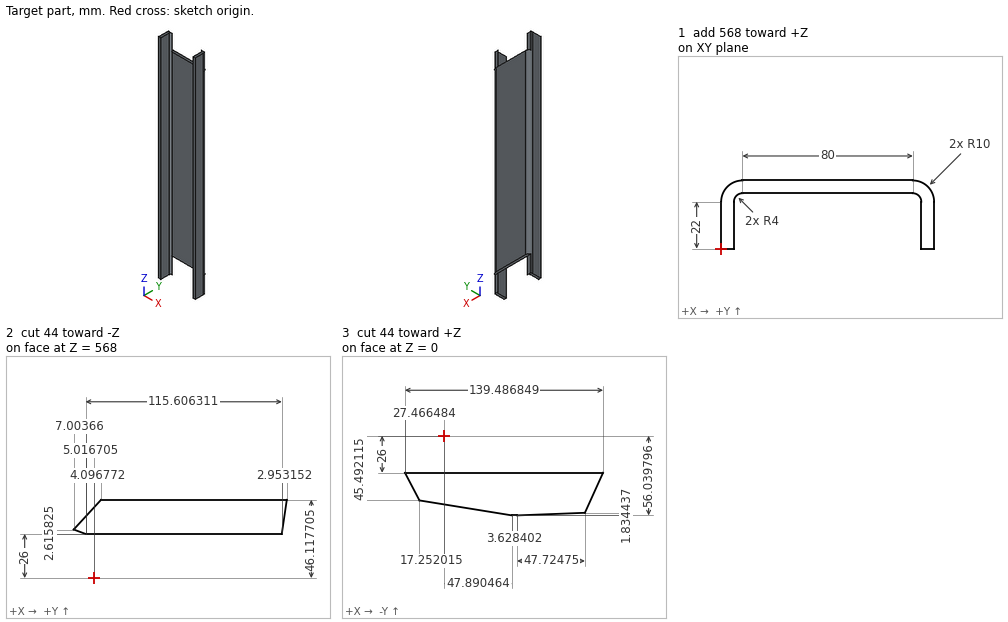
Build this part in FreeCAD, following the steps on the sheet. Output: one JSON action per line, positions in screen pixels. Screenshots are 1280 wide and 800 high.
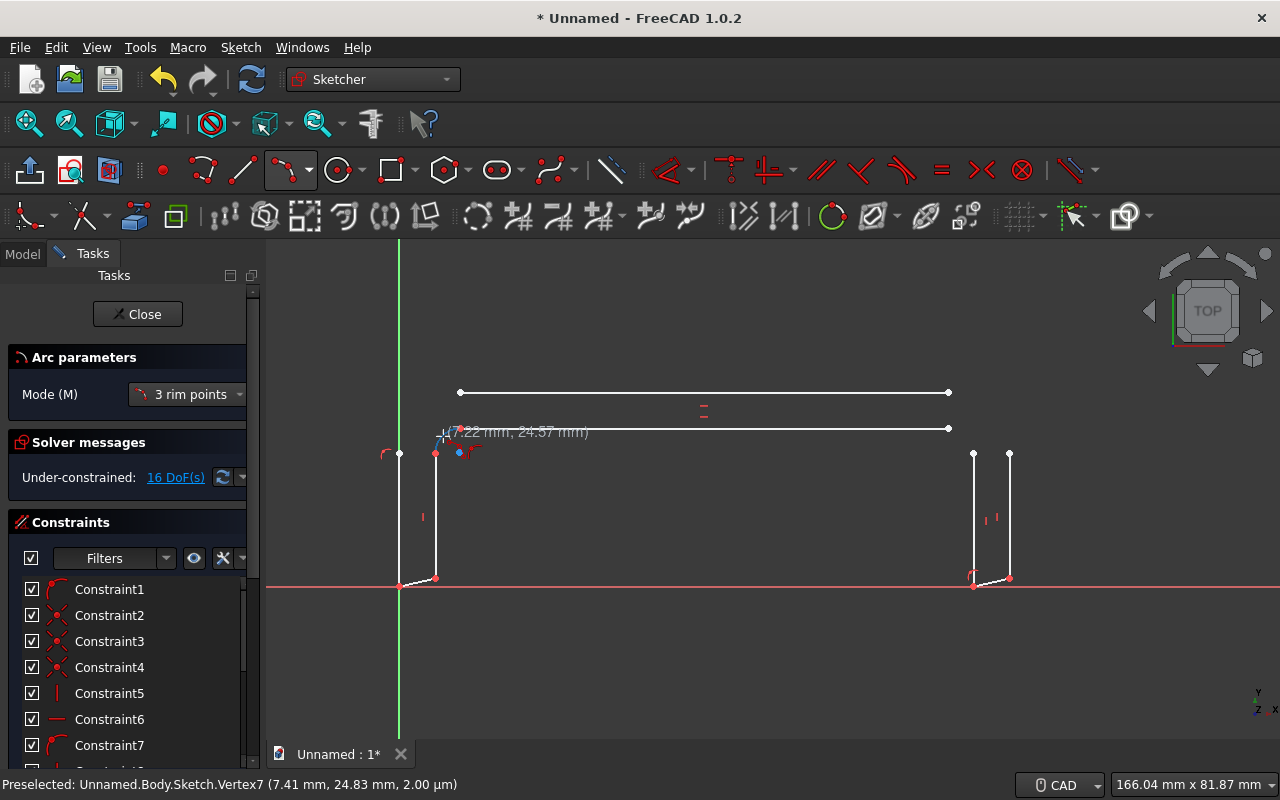
{"action": "left_click", "coordinate": [949, 429]}
{"action": "left_click", "coordinate": [974, 454]}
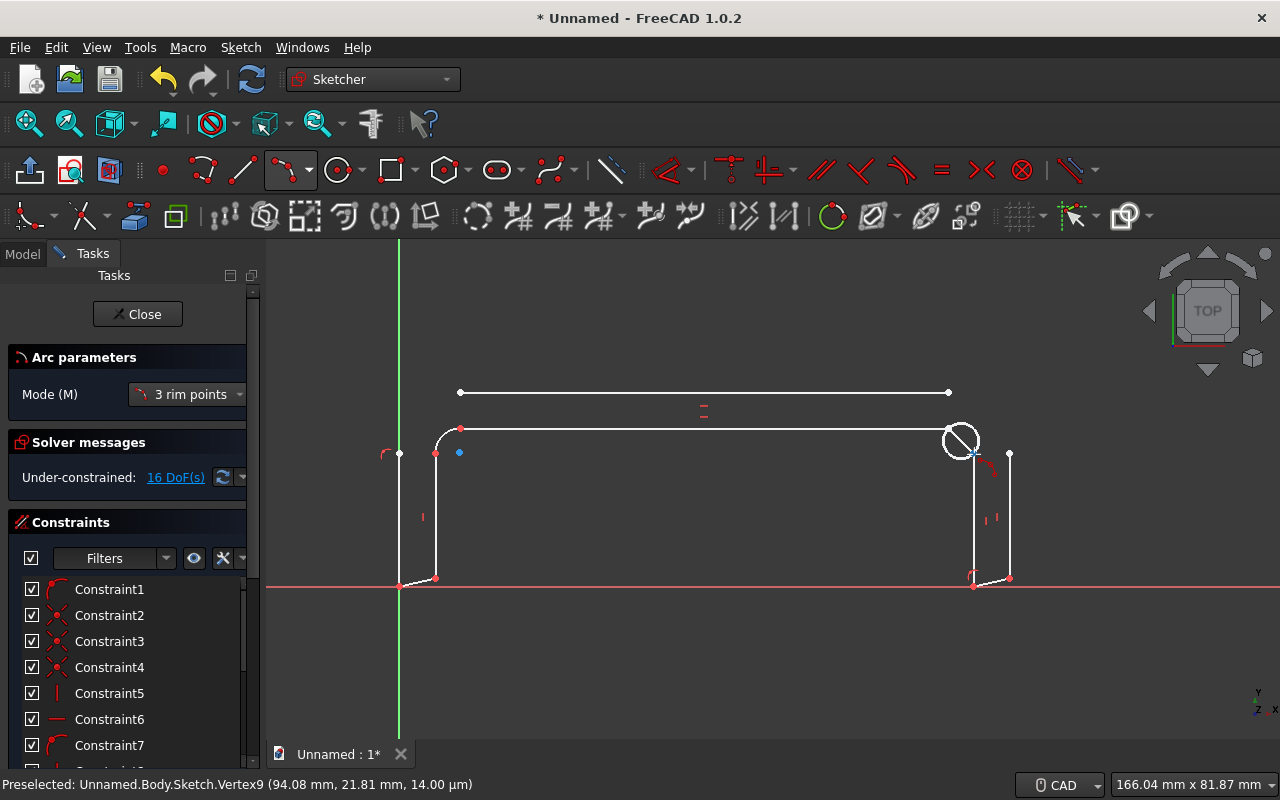
{"action": "scroll", "coordinate": [966, 435], "scroll_direction": "up", "scroll_amount": 4}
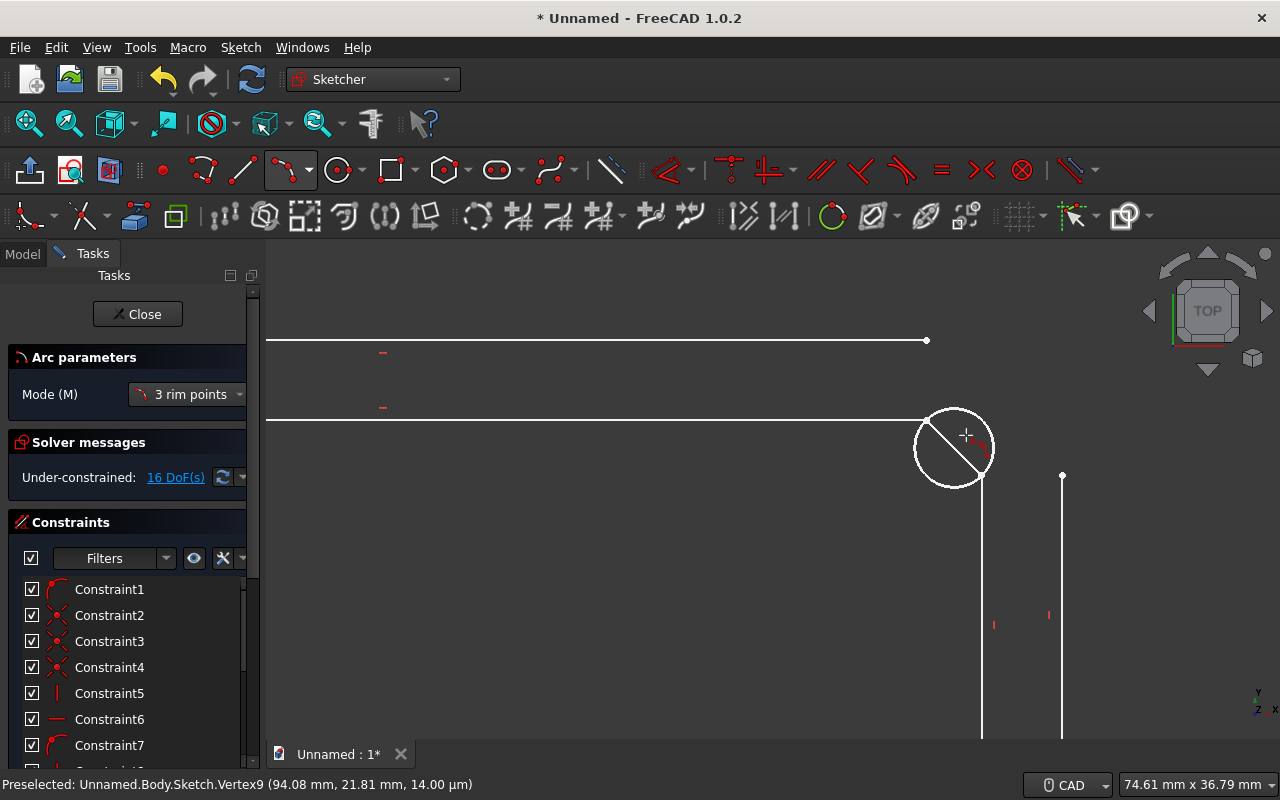
{"action": "left_click", "coordinate": [965, 435]}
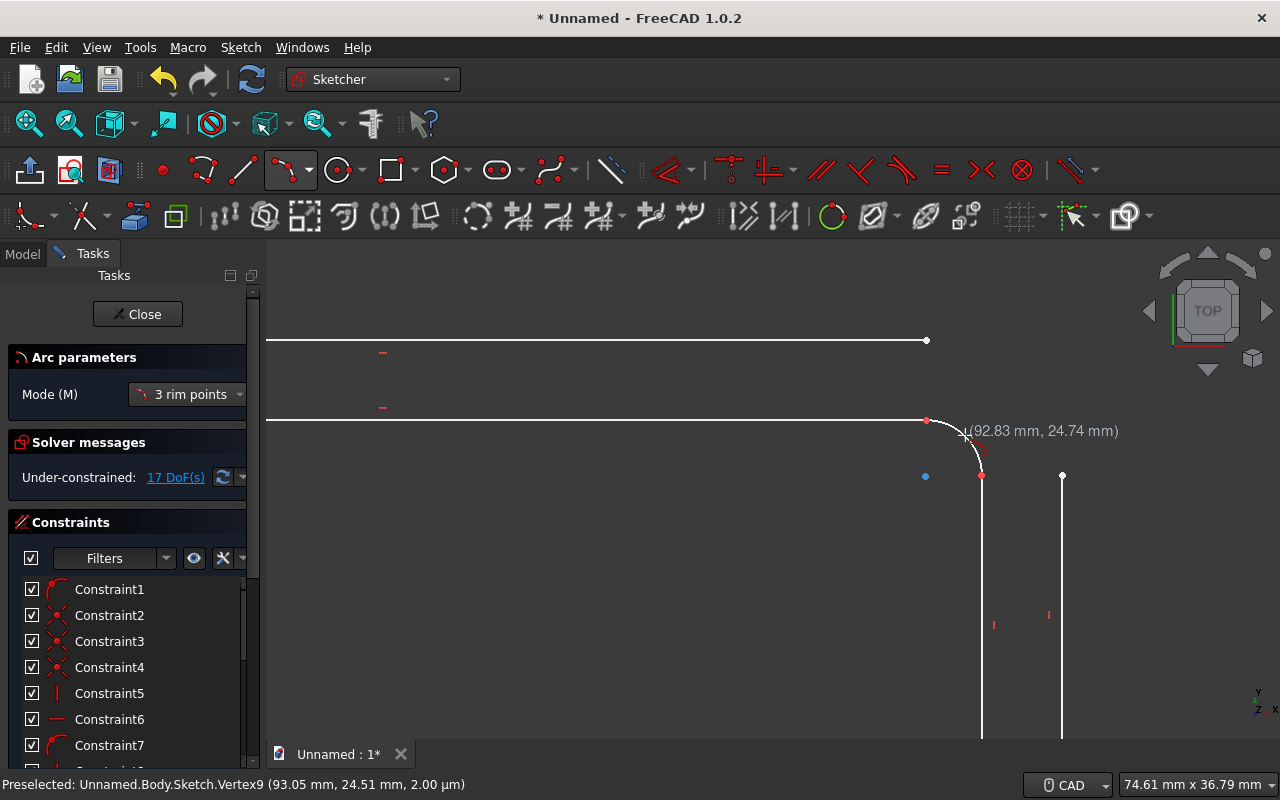
{"action": "left_click", "coordinate": [1062, 476]}
{"action": "left_click", "coordinate": [926, 340]}
{"action": "left_click", "coordinate": [1023, 377]}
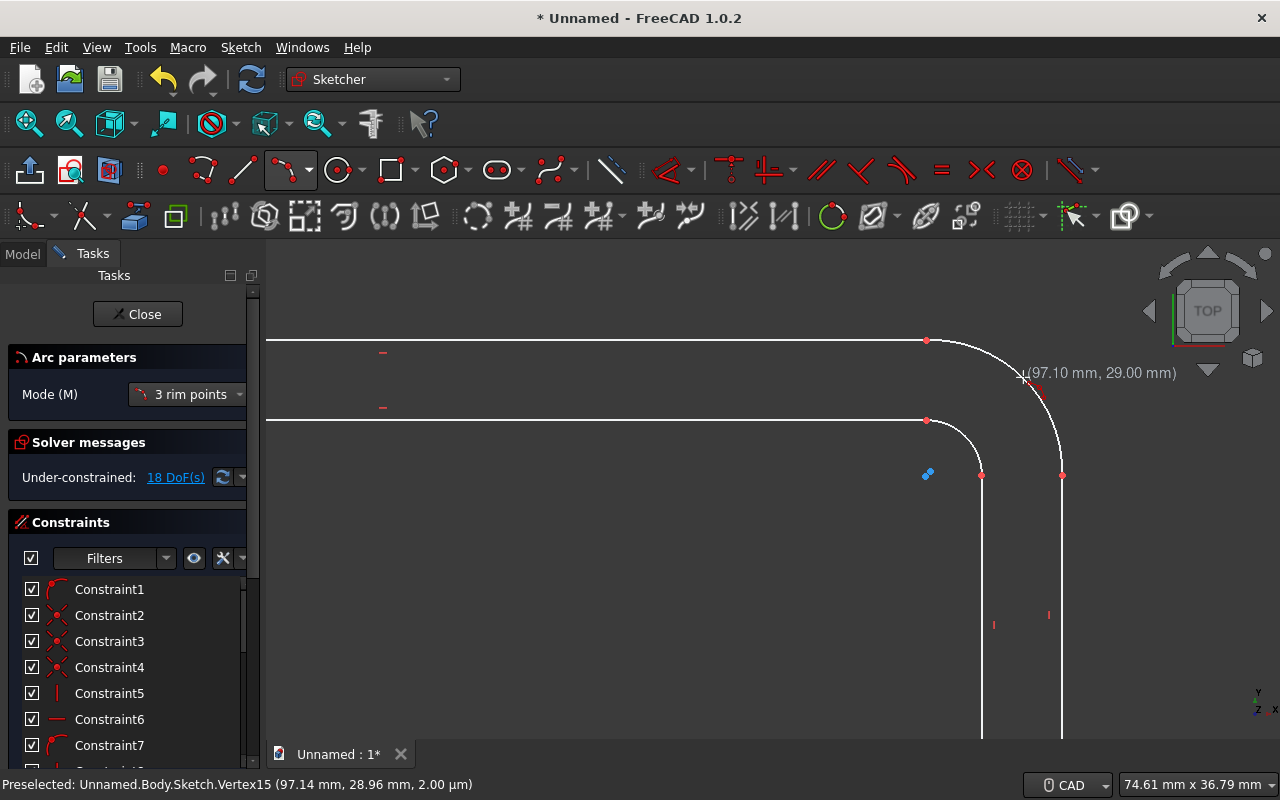
{"action": "scroll", "coordinate": [967, 435], "scroll_direction": "down", "scroll_amount": 4}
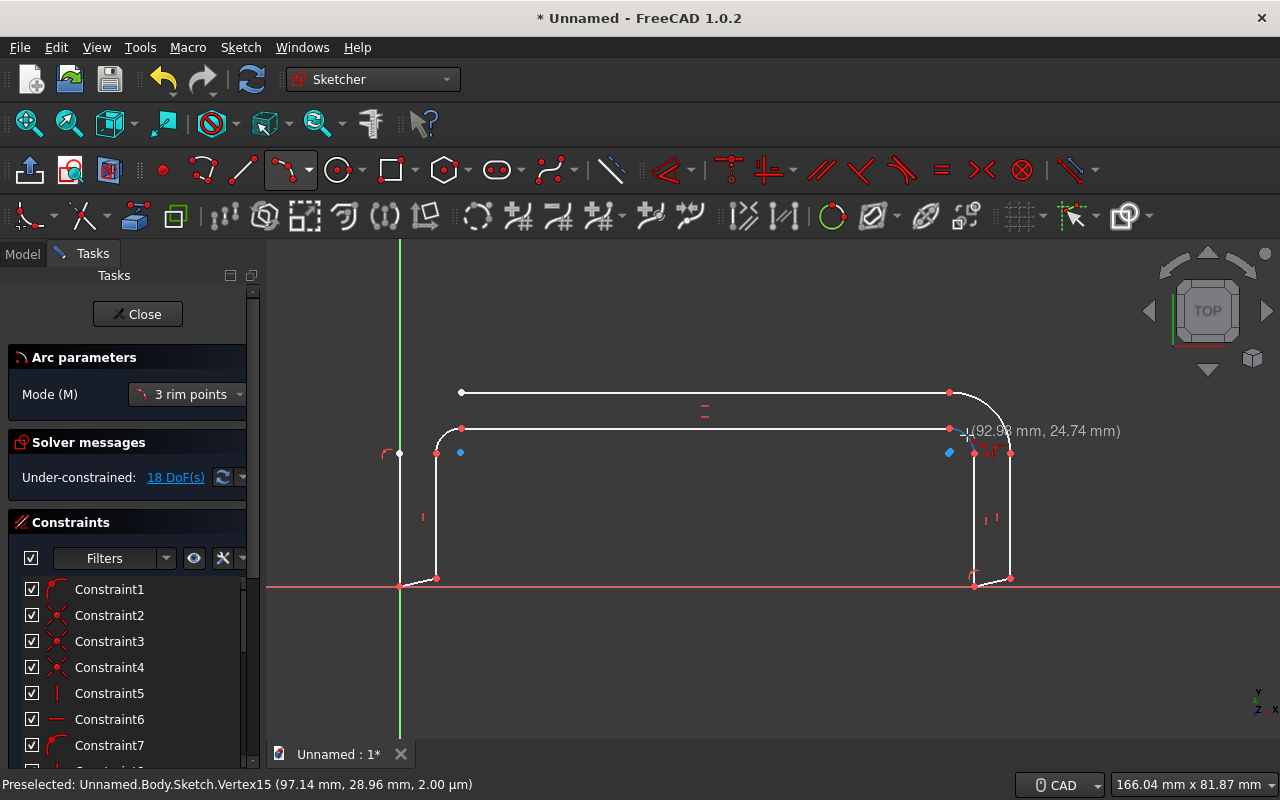
{"action": "left_click", "coordinate": [461, 393]}
{"action": "left_click", "coordinate": [400, 454]}
{"action": "left_click", "coordinate": [417, 409]}
{"action": "key", "text": "Escape"}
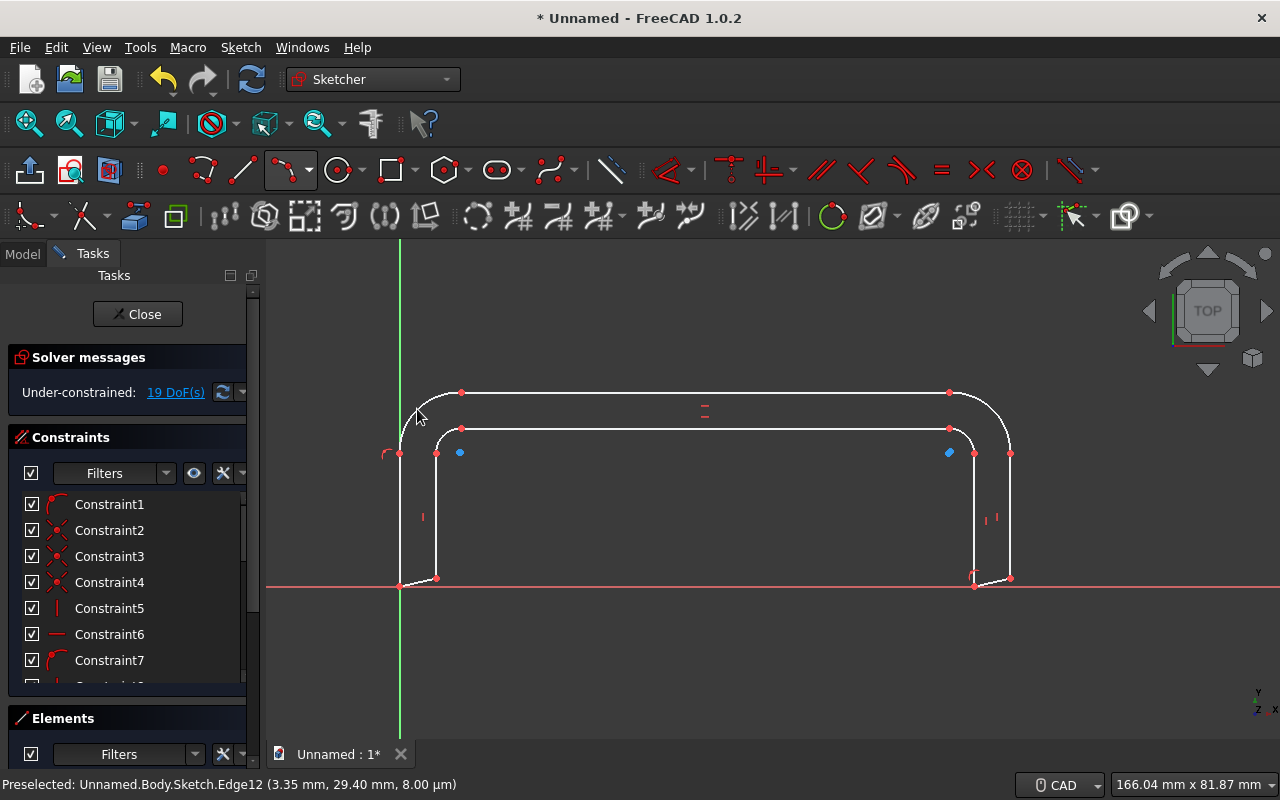
{"action": "left_click", "coordinate": [400, 494]}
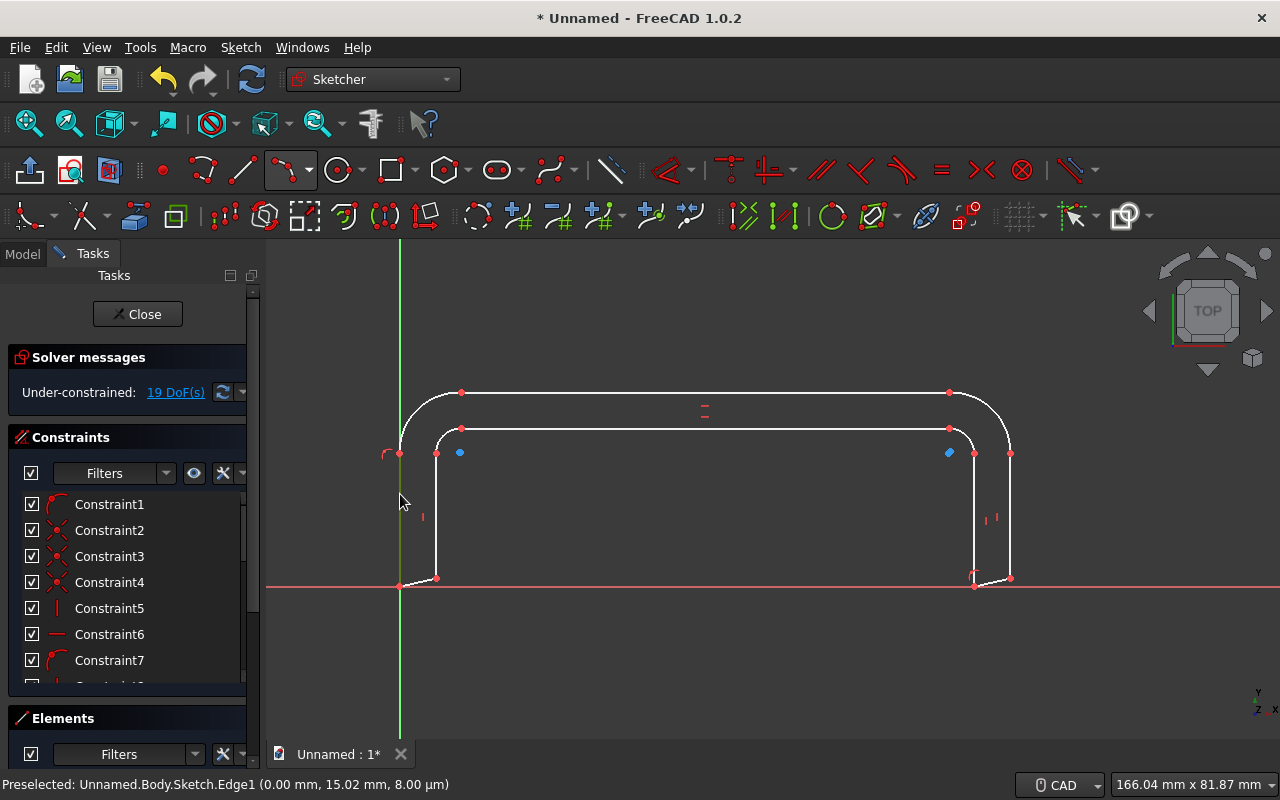
{"action": "left_click", "coordinate": [433, 399]}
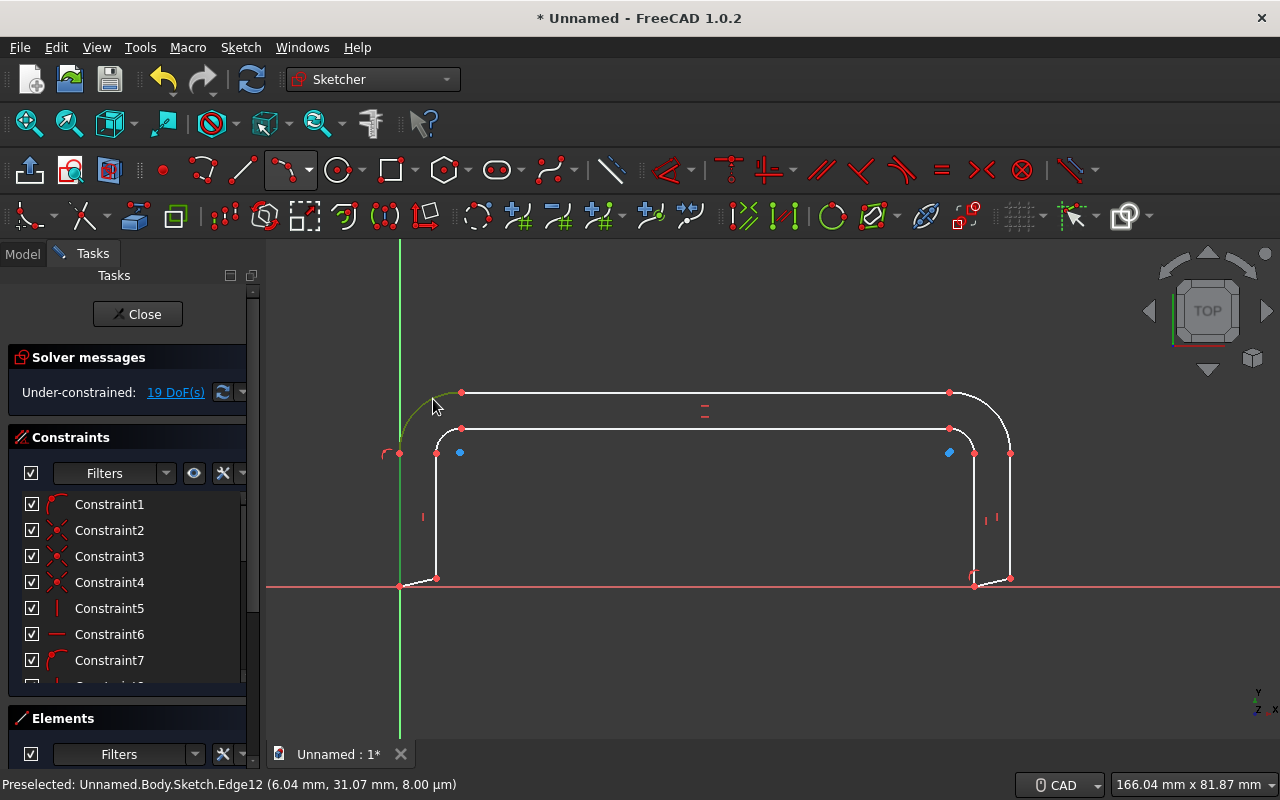
{"action": "left_click", "coordinate": [902, 170]}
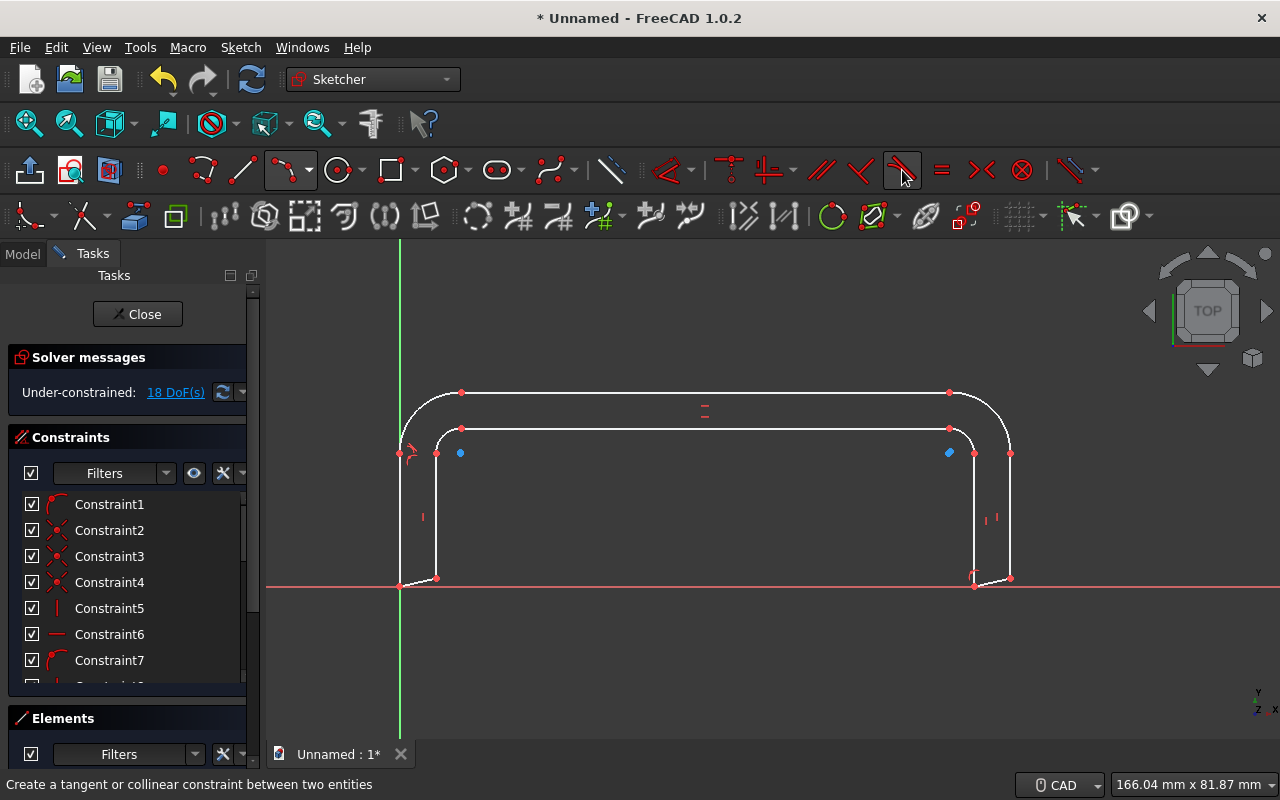
{"action": "left_click", "coordinate": [436, 541]}